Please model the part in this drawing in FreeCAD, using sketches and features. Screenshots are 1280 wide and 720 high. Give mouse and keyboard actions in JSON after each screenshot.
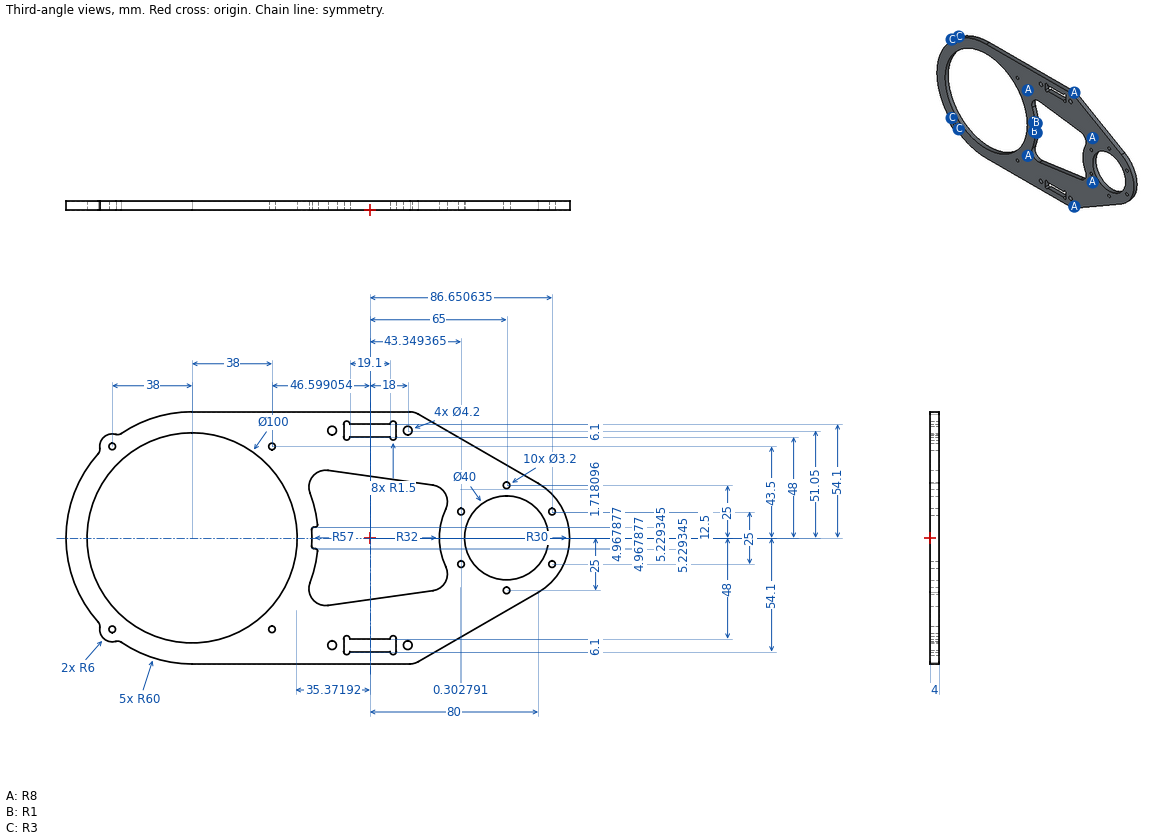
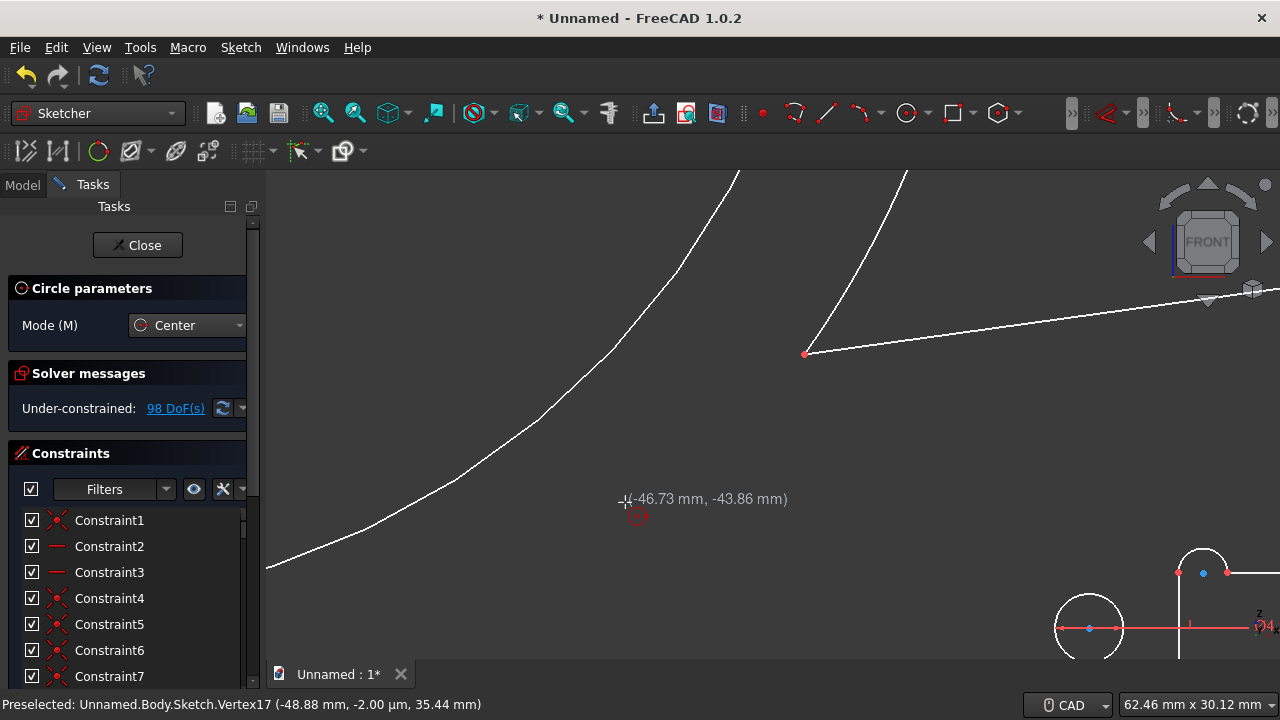
{"action": "scroll", "coordinate": [661, 512], "scroll_direction": "down", "scroll_amount": 10}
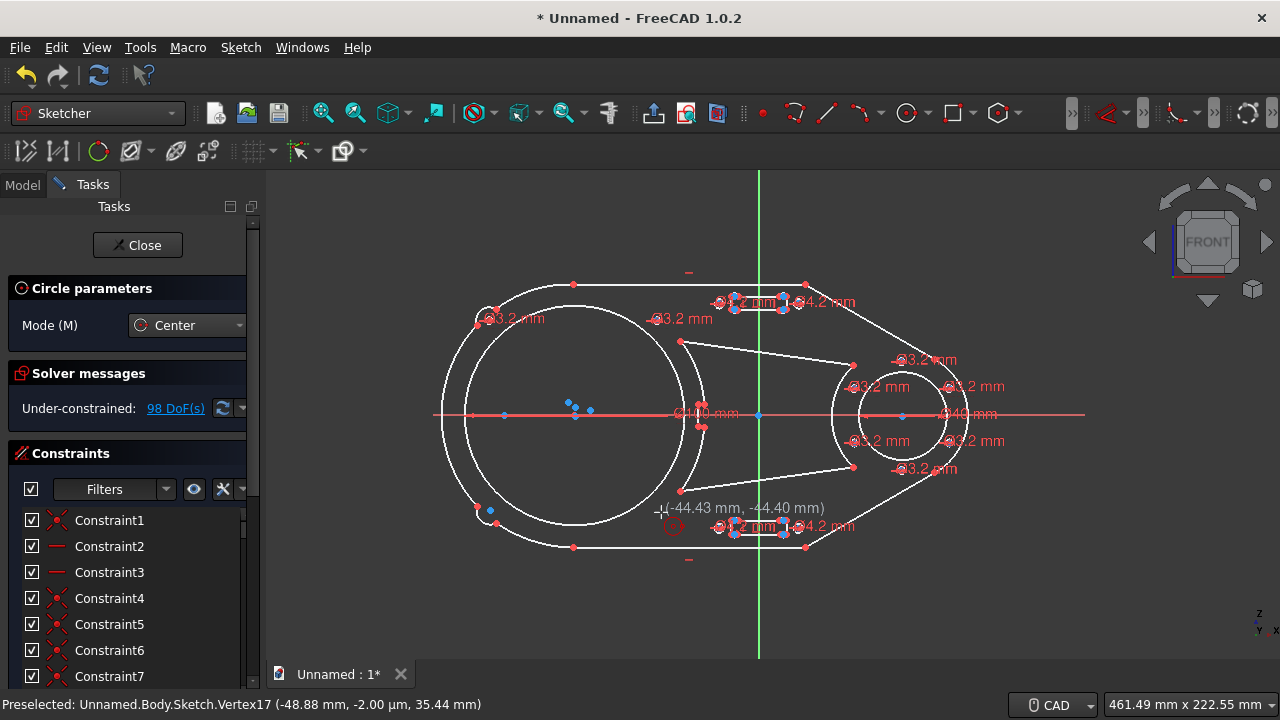
{"action": "left_click", "coordinate": [657, 511]}
{"action": "mouse_move", "coordinate": [659, 508]}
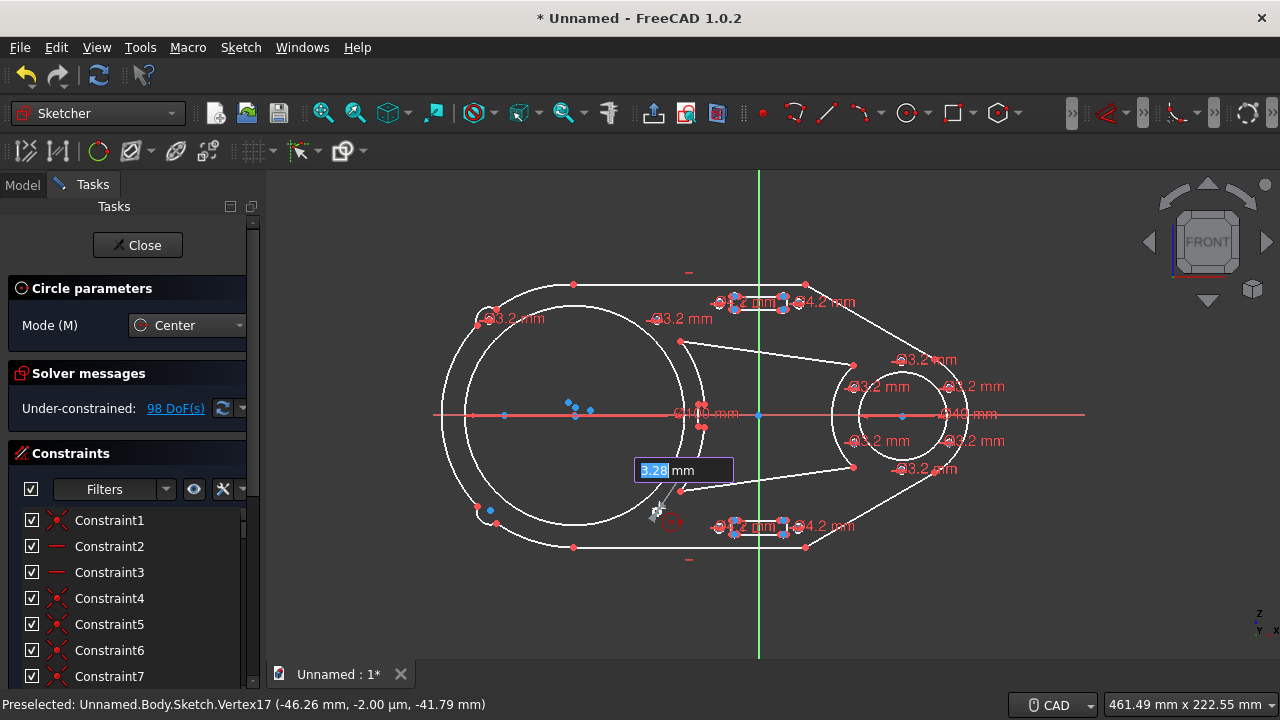
{"action": "type", "text": "3.2"}
{"action": "key", "text": "Return"}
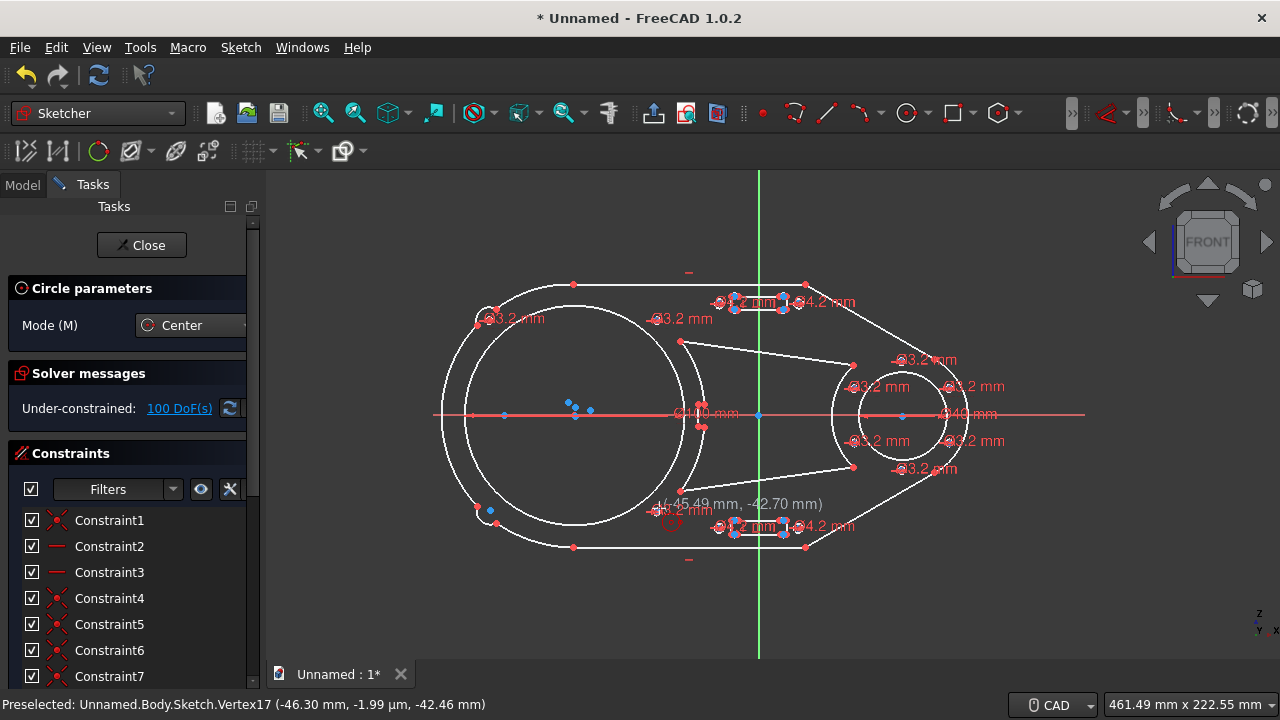
{"action": "scroll", "coordinate": [490, 511], "scroll_direction": "up", "scroll_amount": 10}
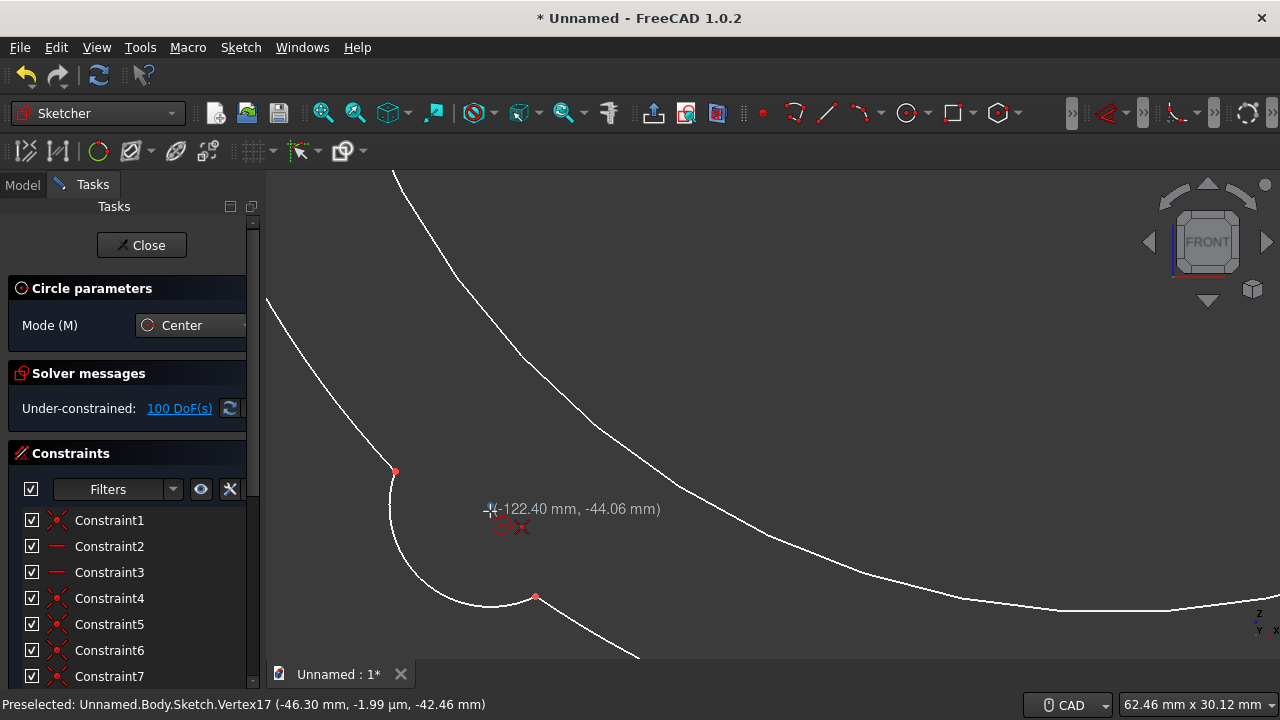
{"action": "scroll", "coordinate": [490, 511], "scroll_direction": "down", "scroll_amount": 10}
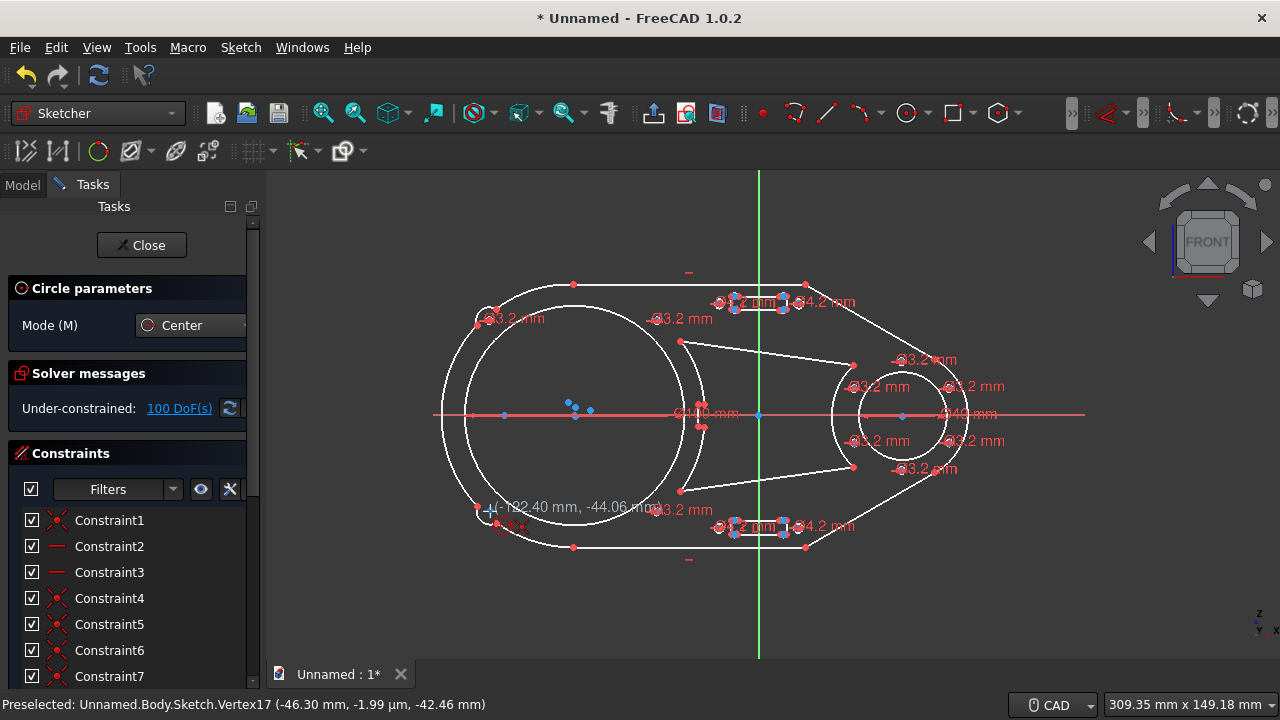
{"action": "left_click", "coordinate": [490, 511]}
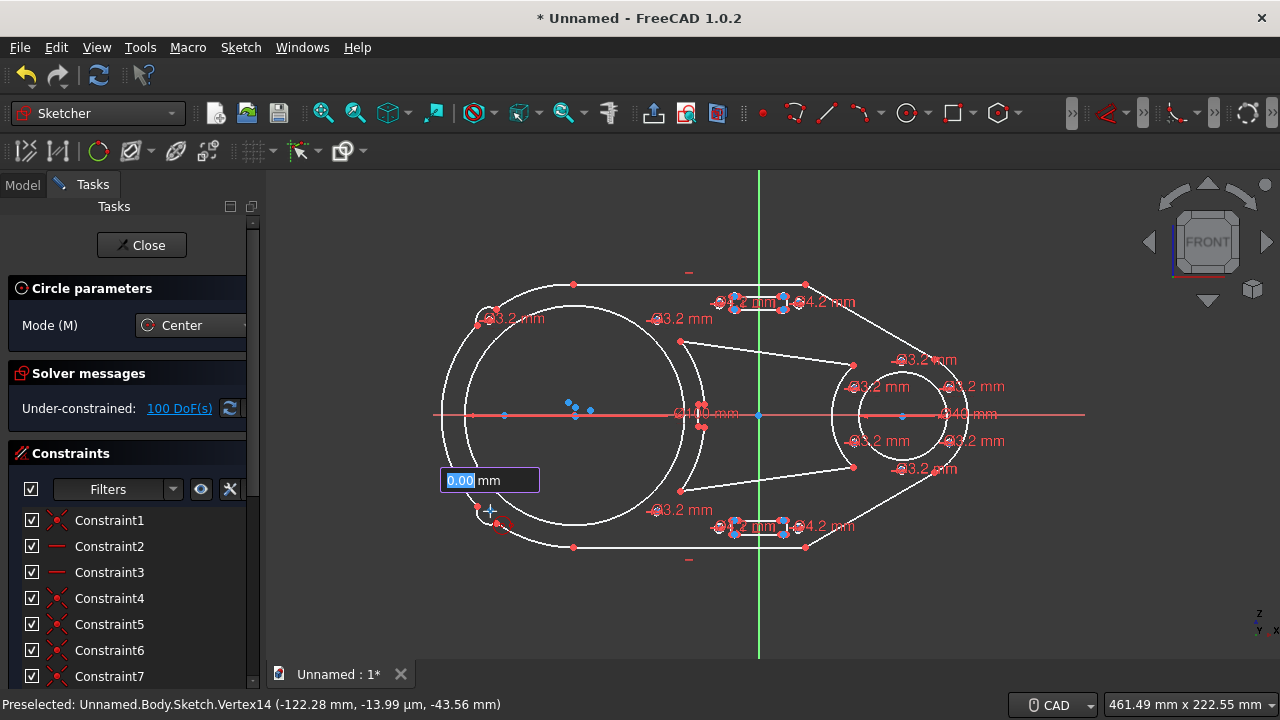
{"action": "scroll", "coordinate": [493, 510], "scroll_direction": "up", "scroll_amount": 8}
{"action": "mouse_move", "coordinate": [491, 505]}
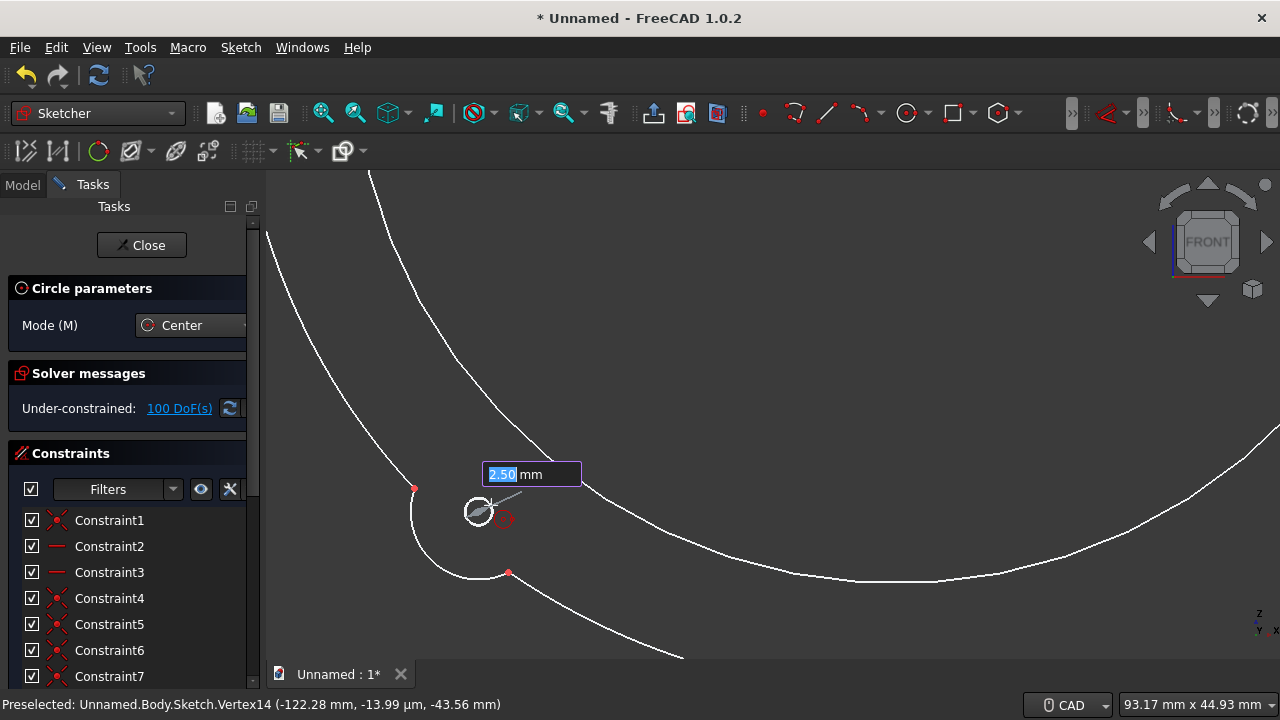
{"action": "type", "text": "3.2"}
{"action": "key", "text": "Return"}
{"action": "key", "text": "Escape"}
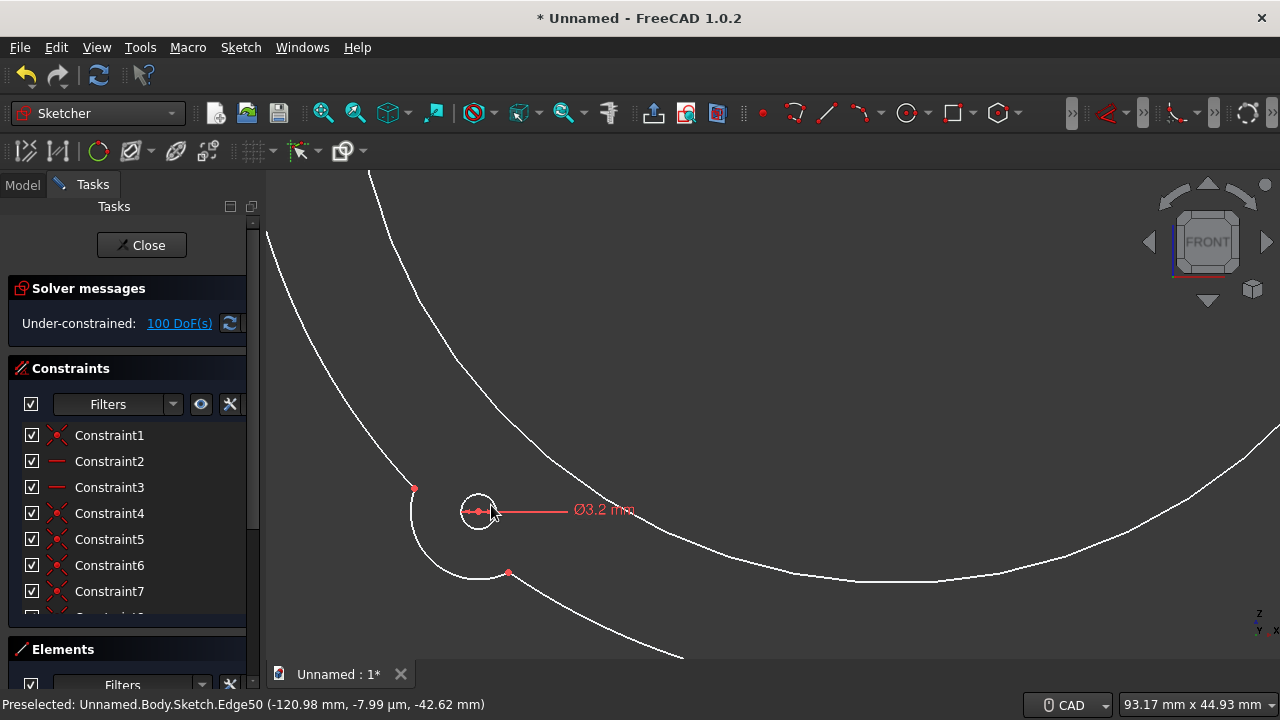
{"action": "scroll", "coordinate": [493, 510], "scroll_direction": "down", "scroll_amount": 8}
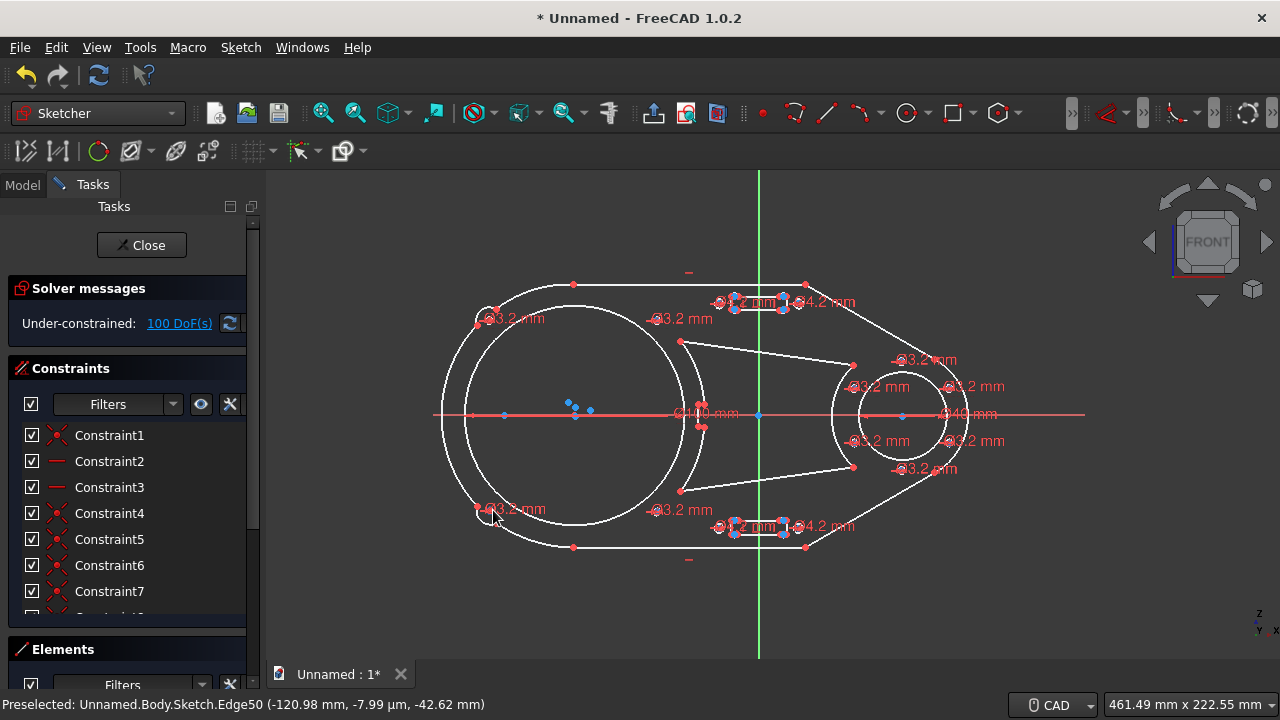
{"action": "left_click", "coordinate": [896, 495]}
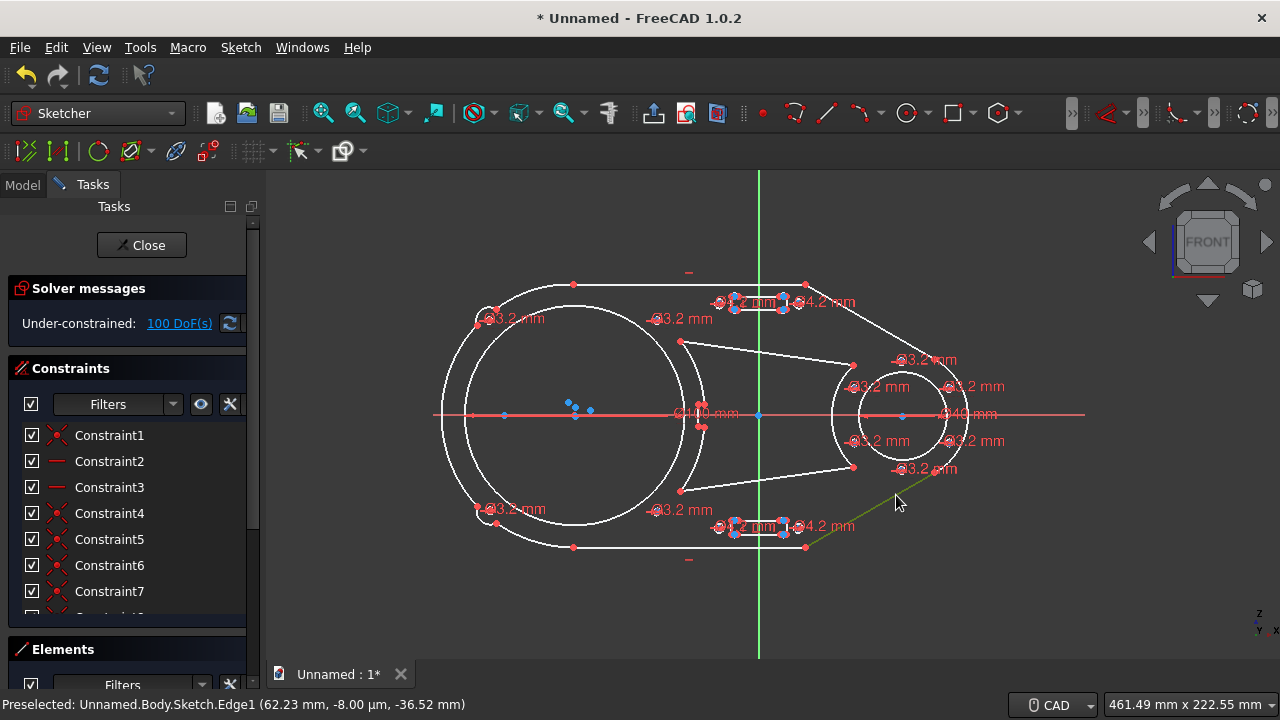
{"action": "scroll", "coordinate": [962, 443], "scroll_direction": "up", "scroll_amount": 2}